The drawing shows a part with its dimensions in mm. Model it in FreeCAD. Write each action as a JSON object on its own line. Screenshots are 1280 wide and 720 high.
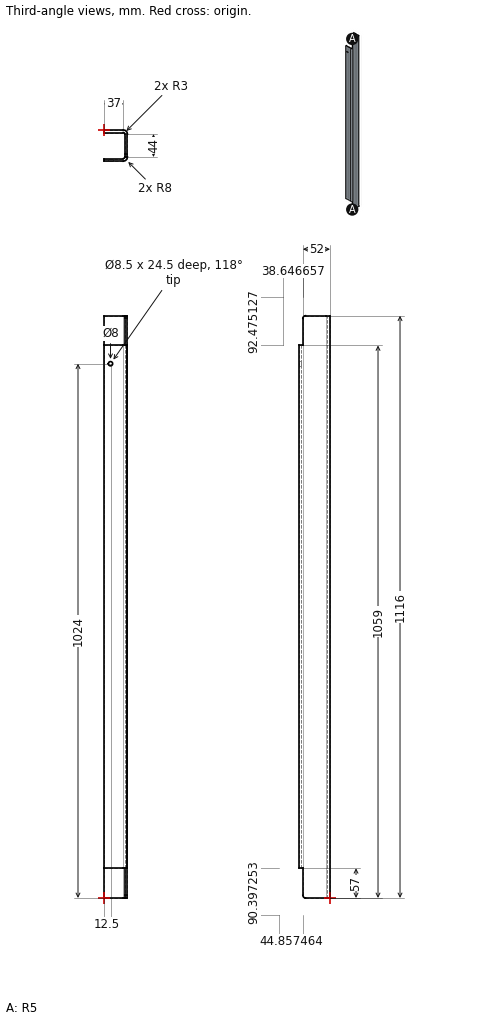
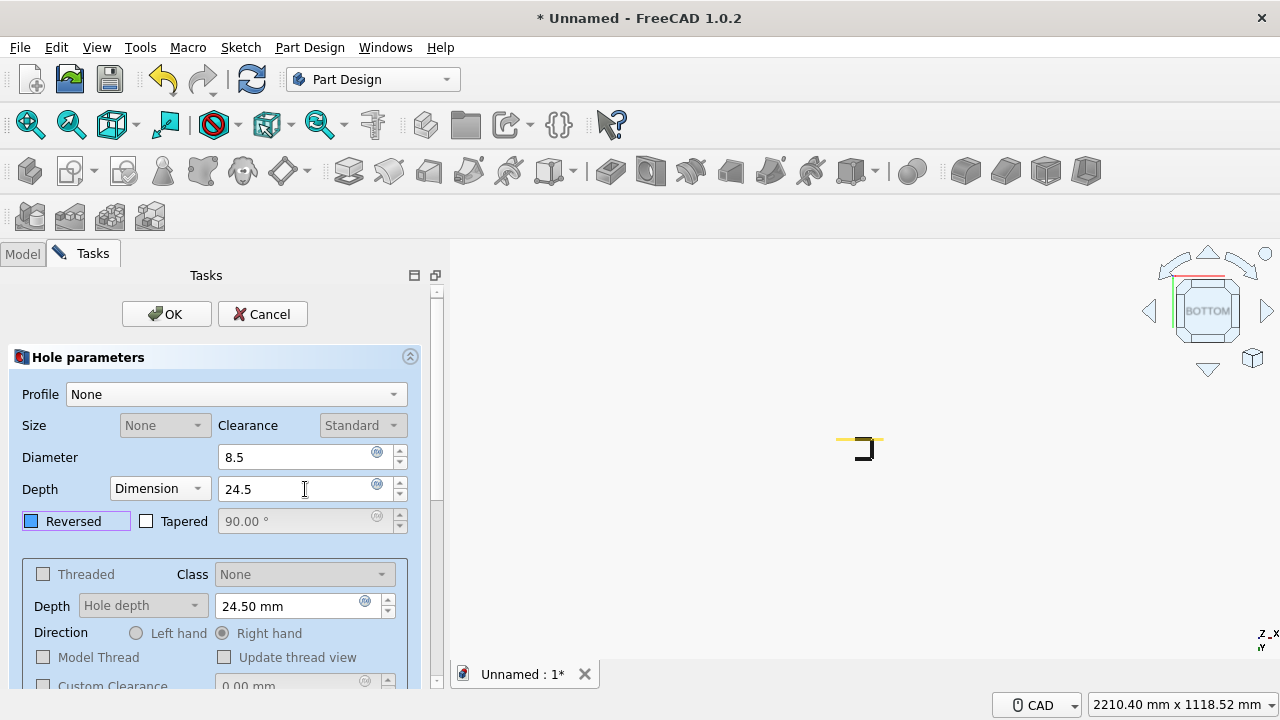
{"action": "left_click", "coordinate": [30, 521]}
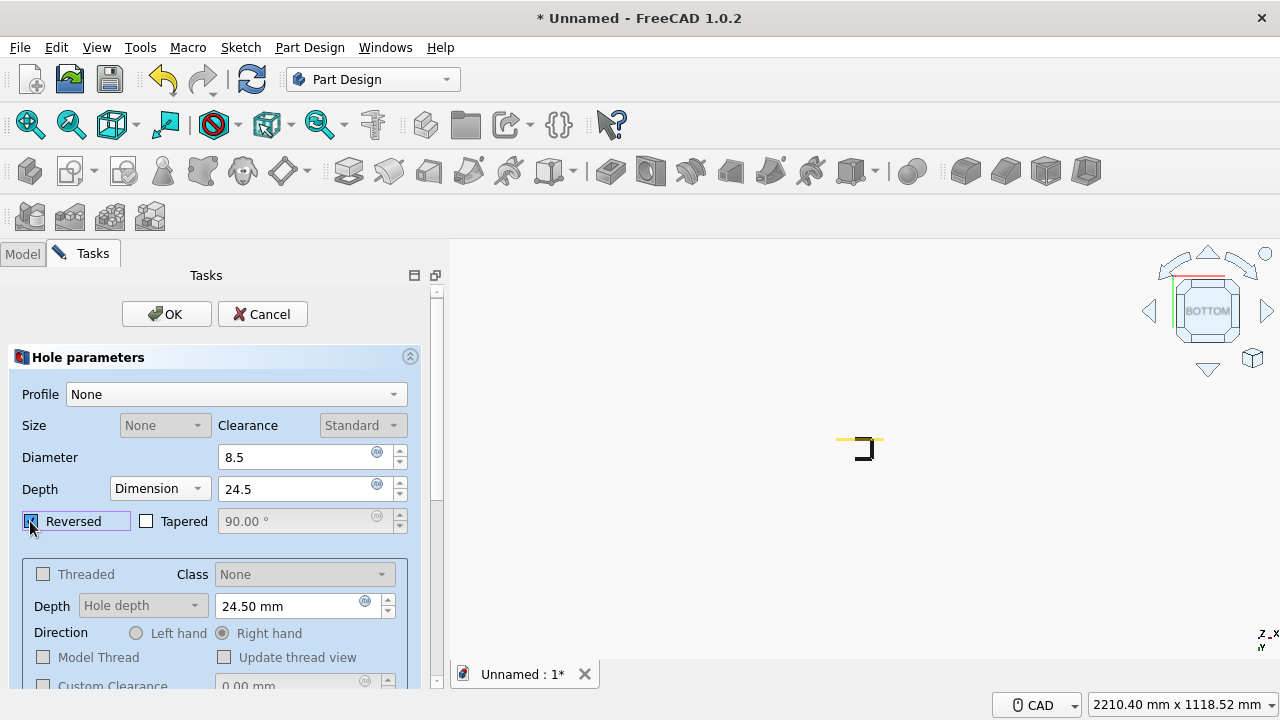
{"action": "left_click", "coordinate": [167, 314]}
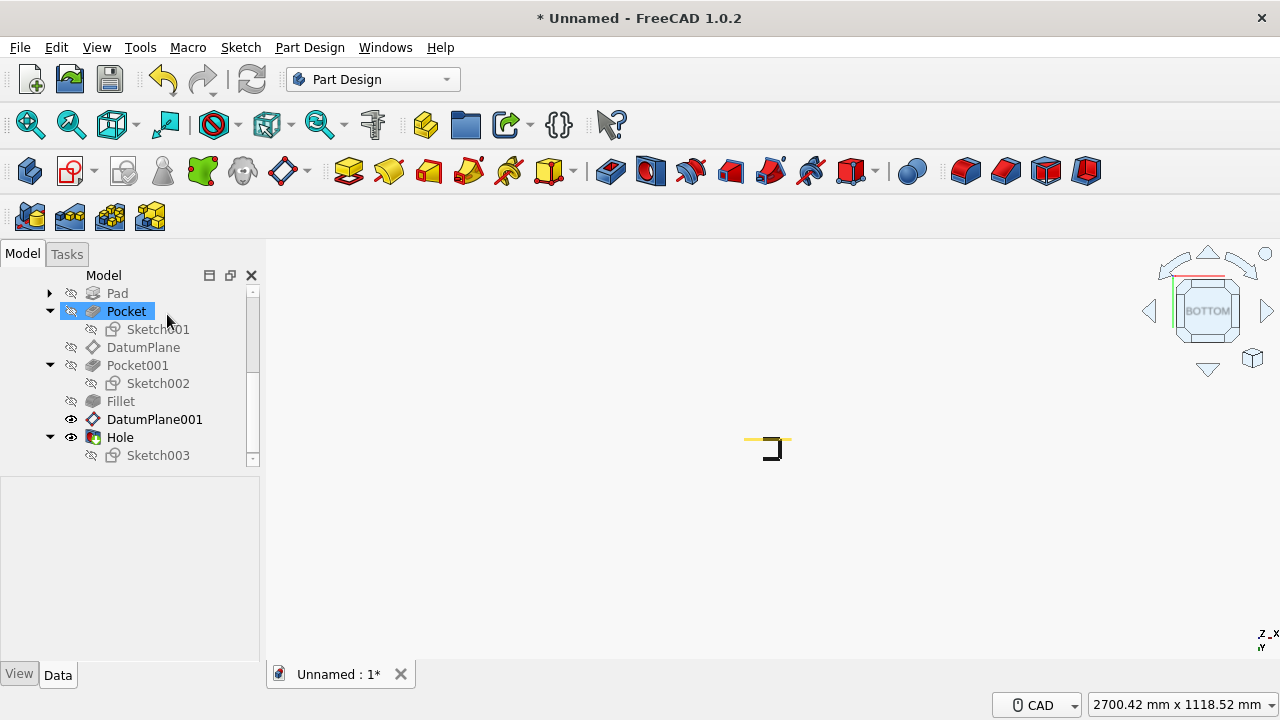
{"action": "left_click", "coordinate": [116, 419]}
{"action": "key", "text": "space"}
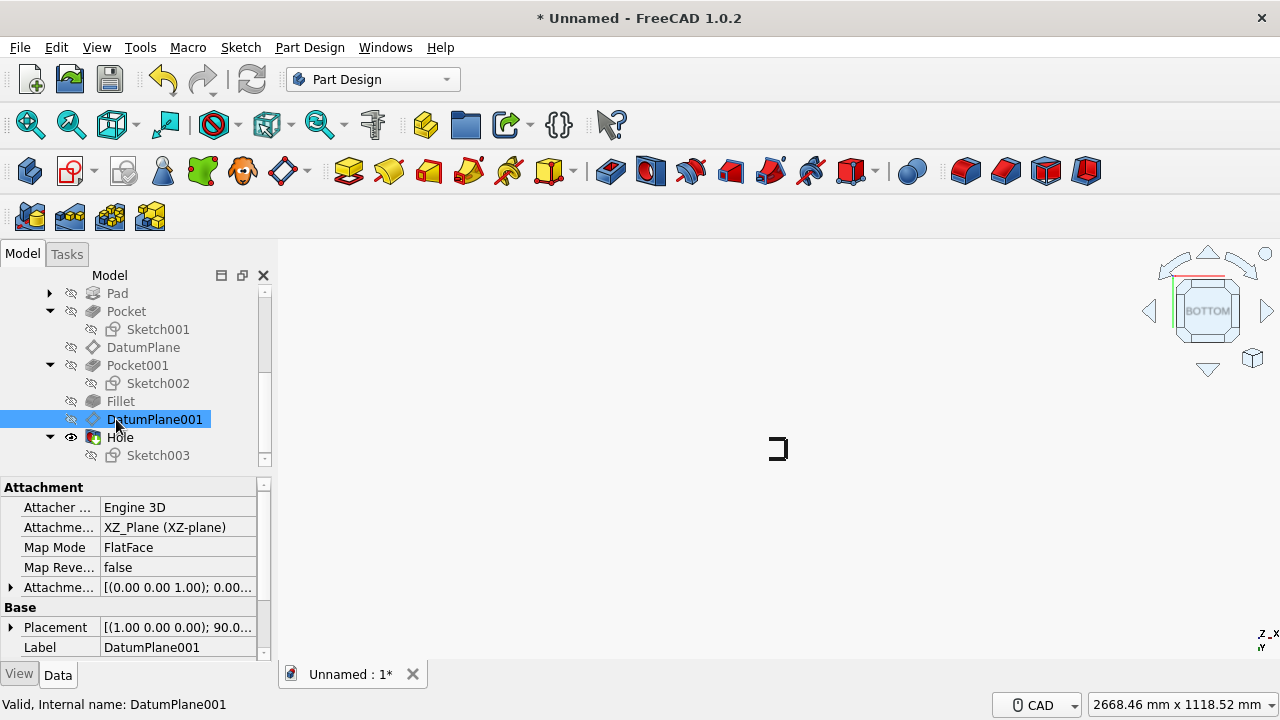
{"action": "key", "text": "0"}